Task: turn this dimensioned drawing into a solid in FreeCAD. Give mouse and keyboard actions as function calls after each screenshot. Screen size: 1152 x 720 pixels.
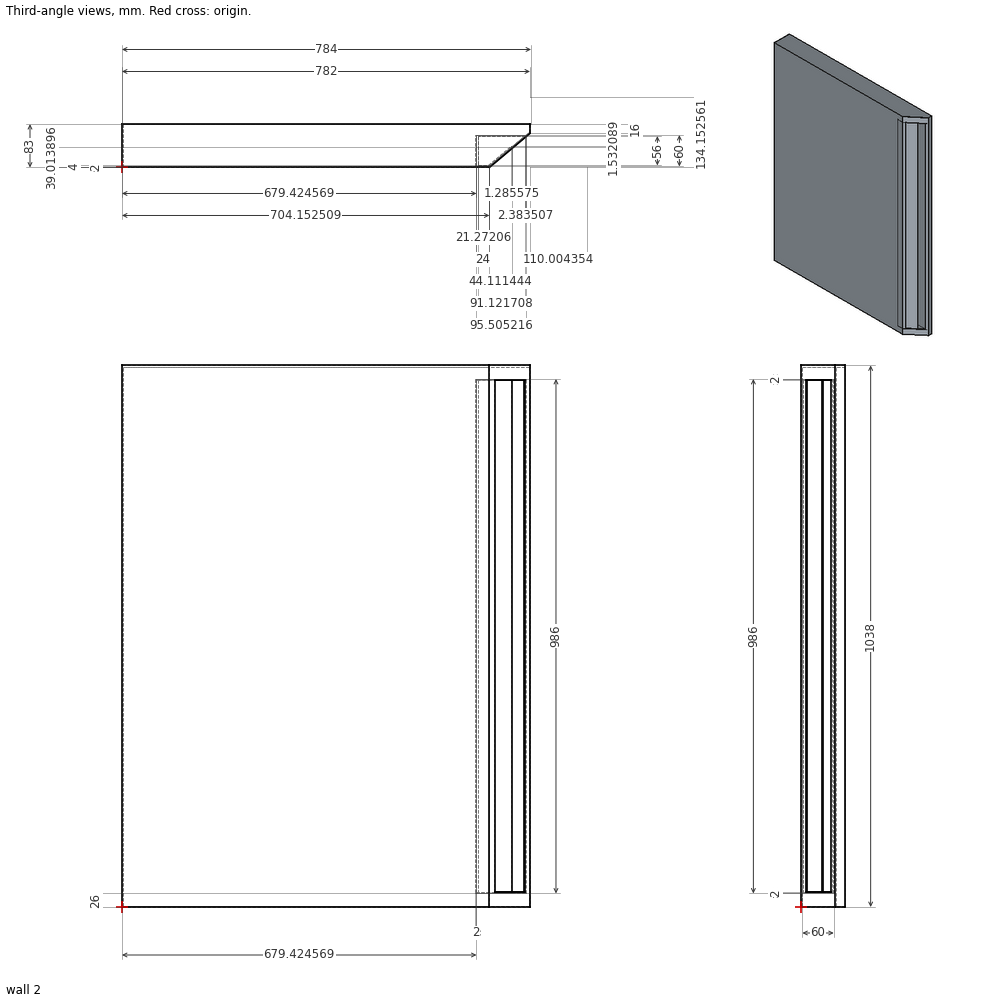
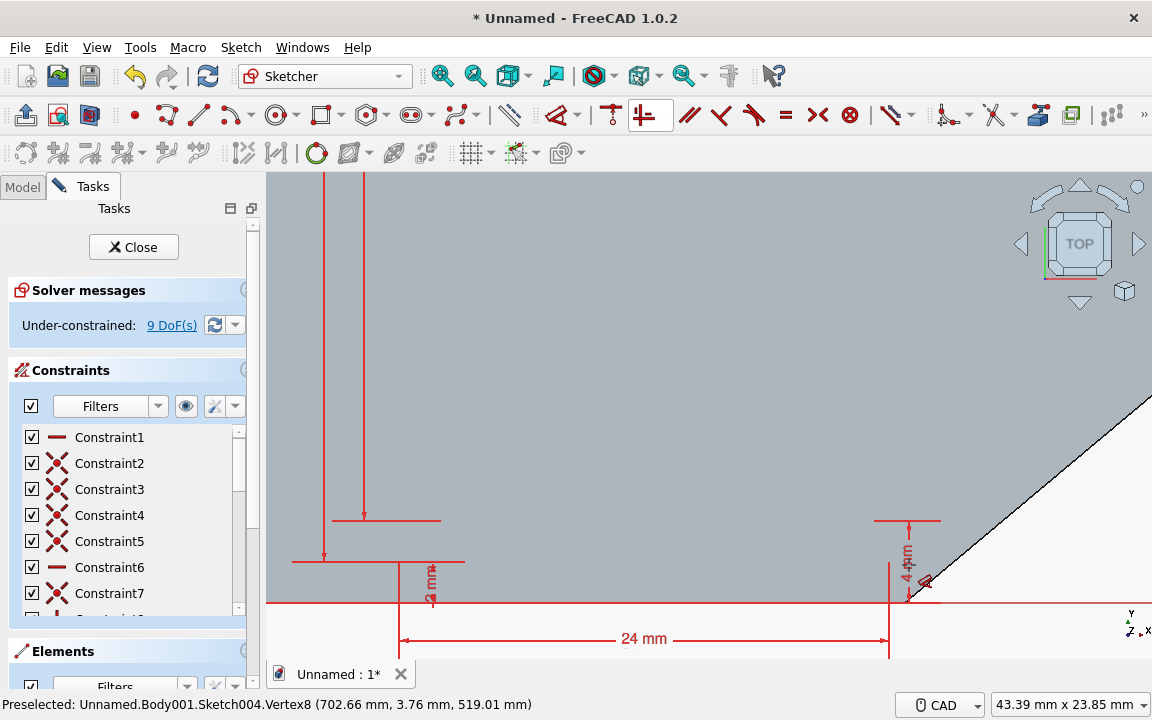
scroll(400, 568, down, 7)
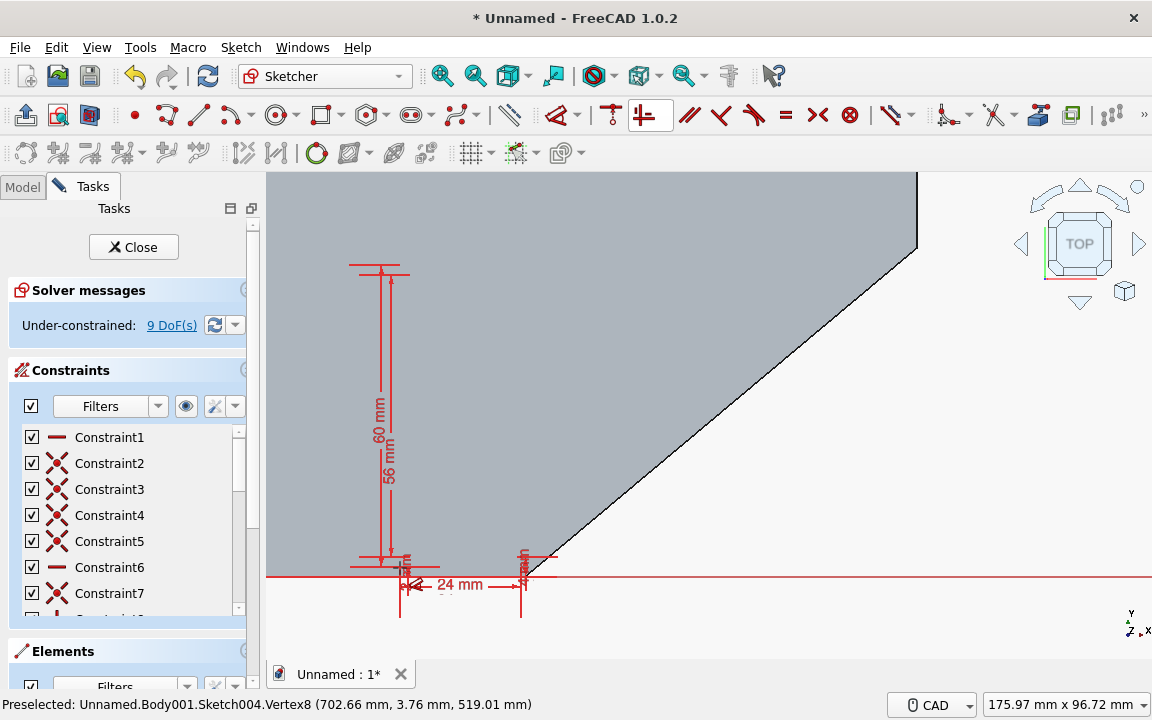
scroll(485, 557, up, 2)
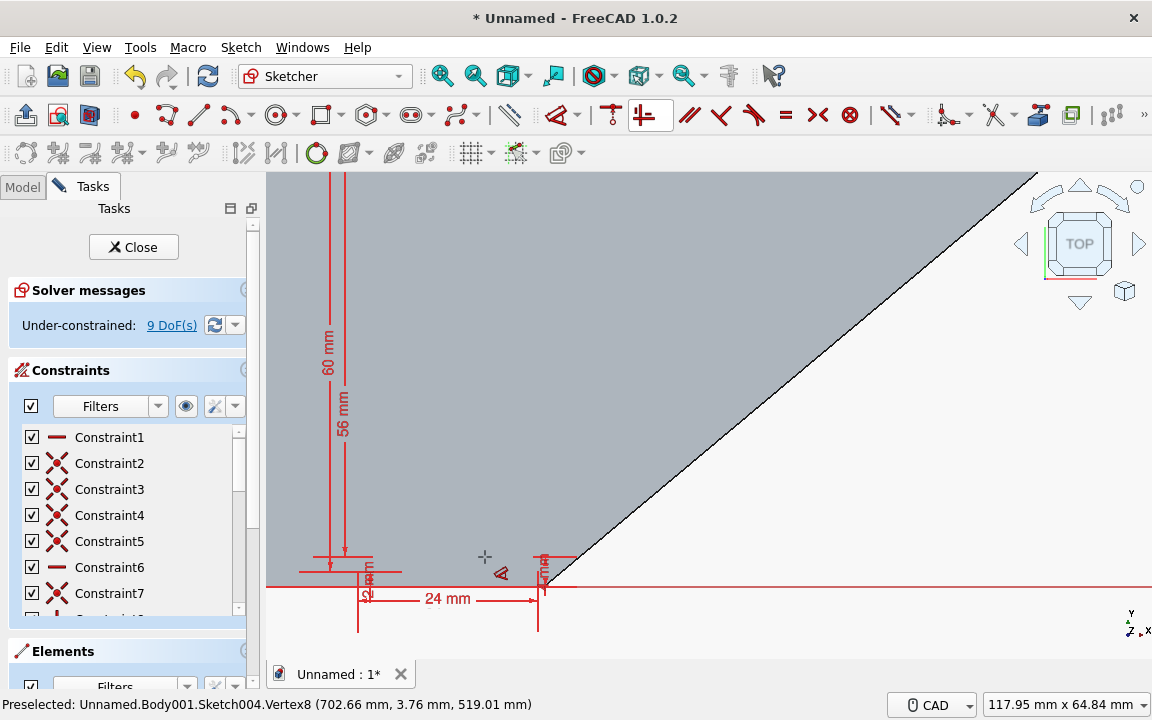
click(485, 557)
click(453, 523)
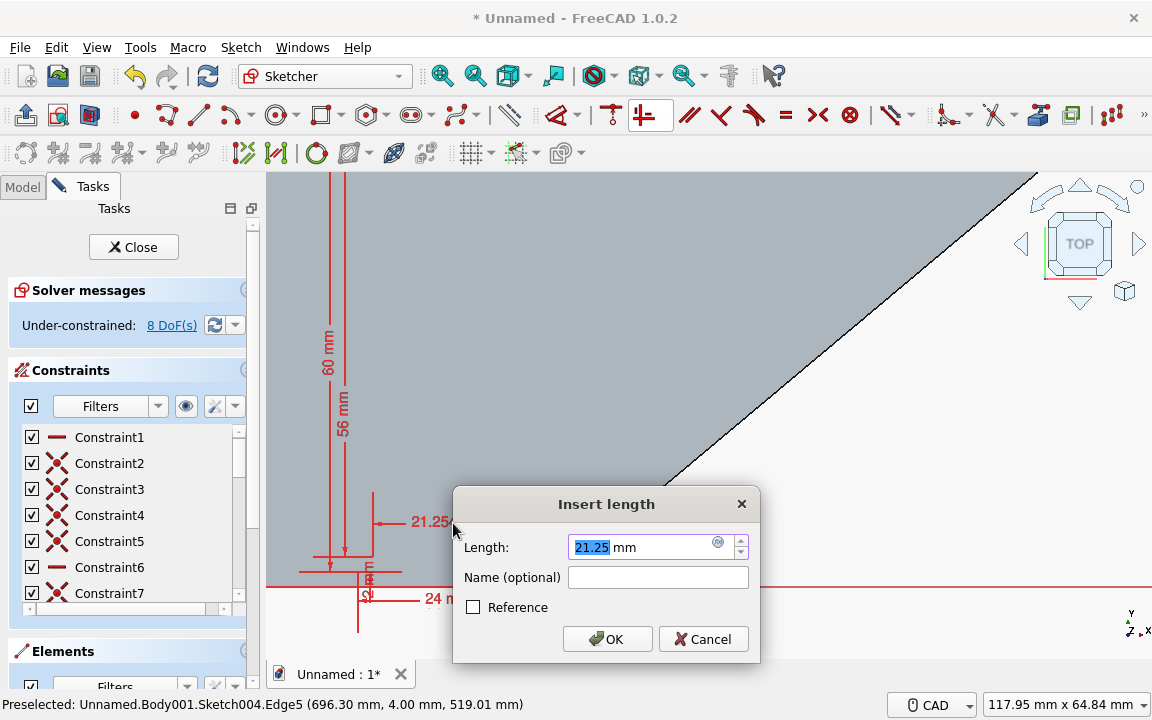
text(21.27206)
key(Return)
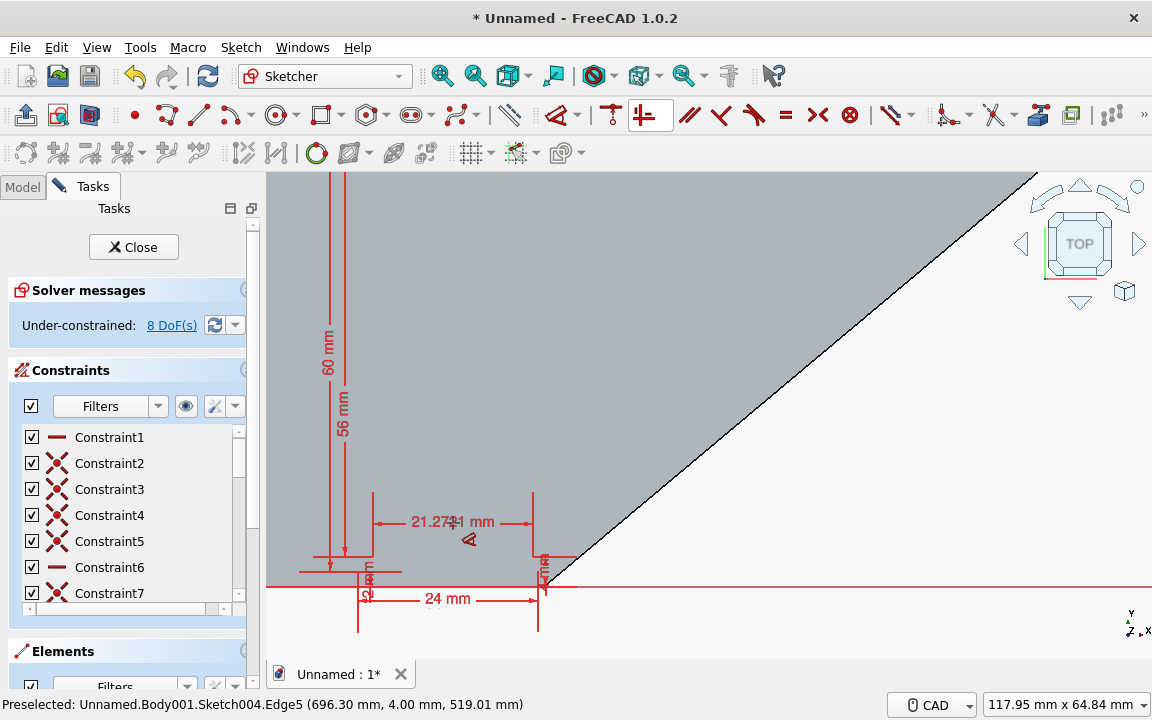
scroll(485, 556, down, 2)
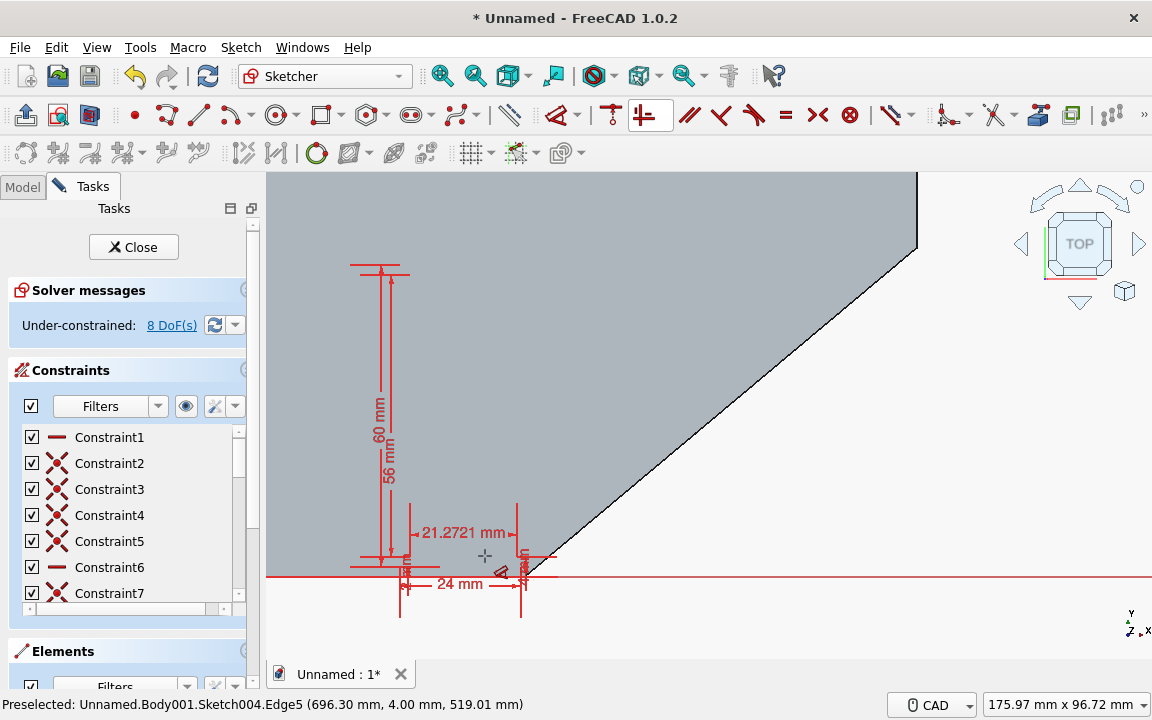
scroll(548, 275, up, 2)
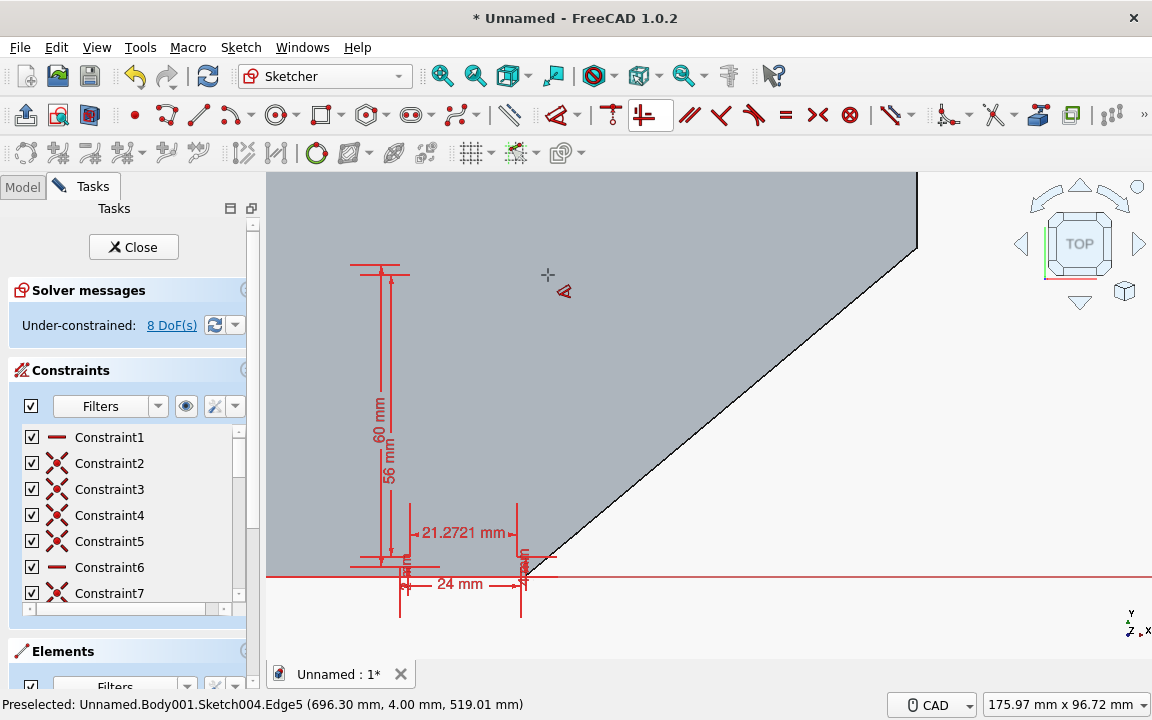
click(548, 275)
click(665, 241)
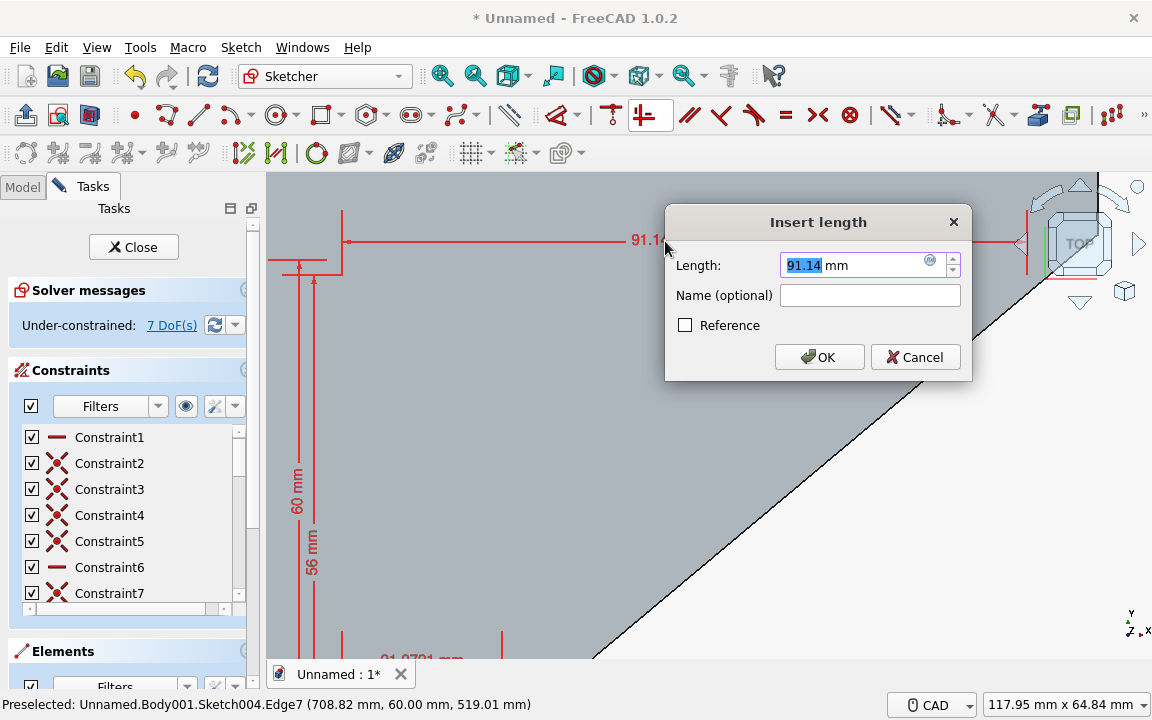
text(91.121708)
key(Return)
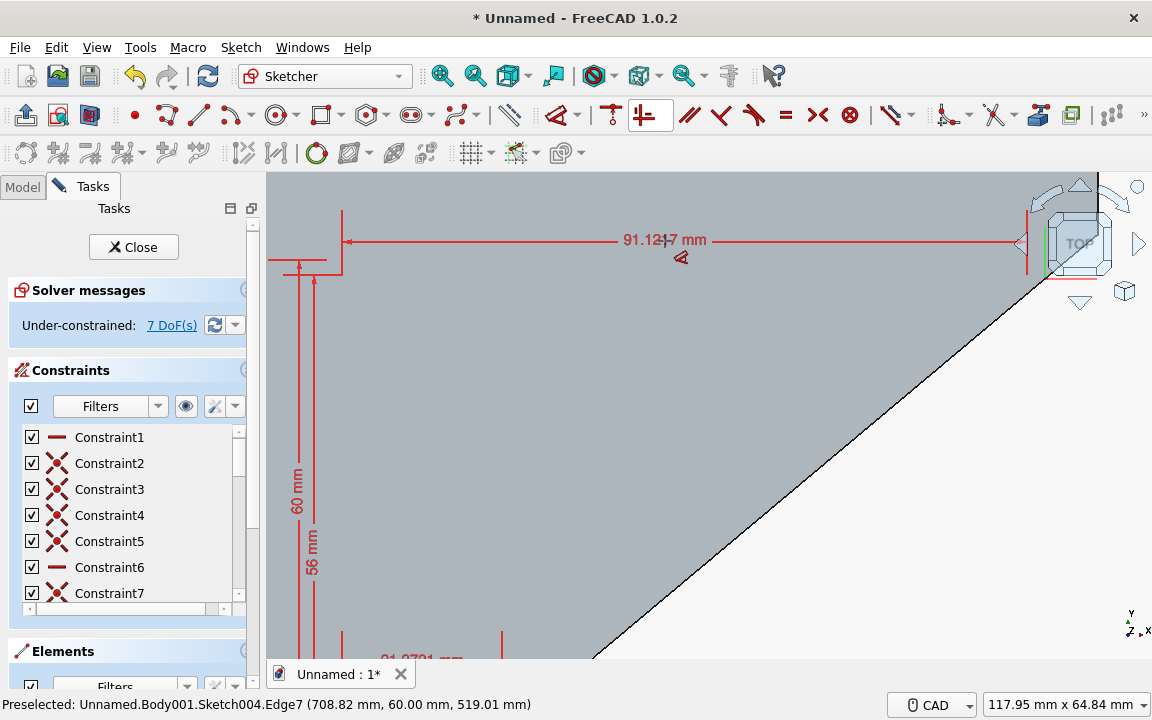
click(829, 260)
click(505, 226)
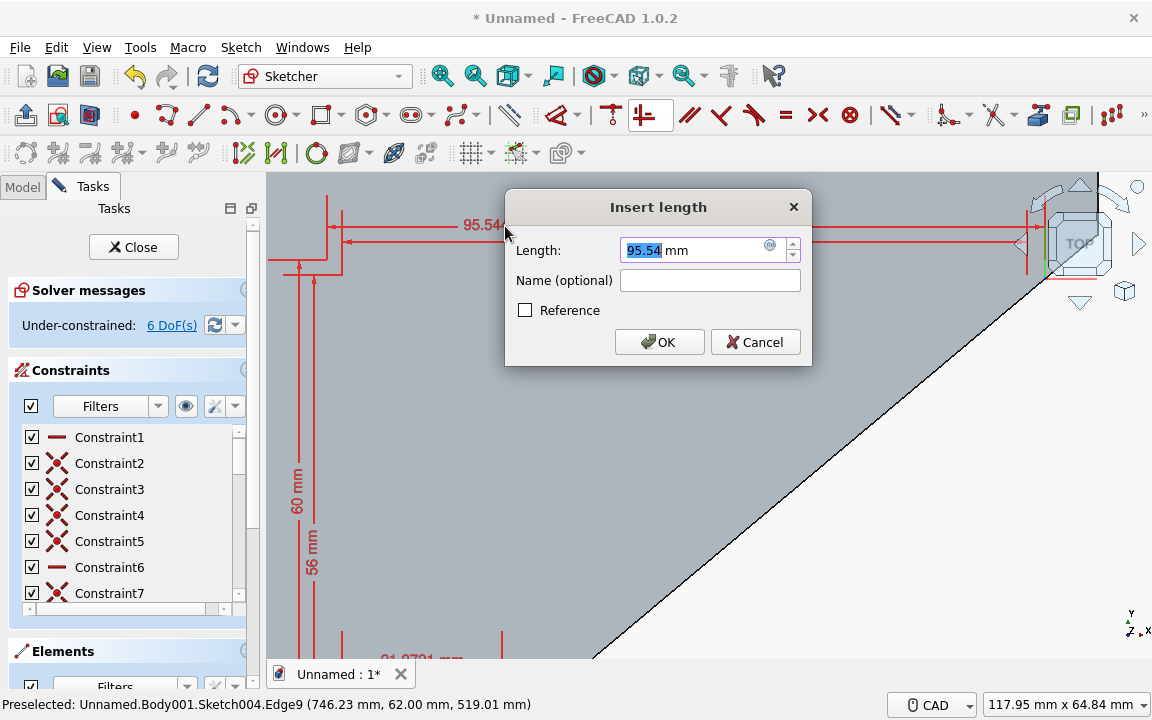
text(95.505216)
key(Return)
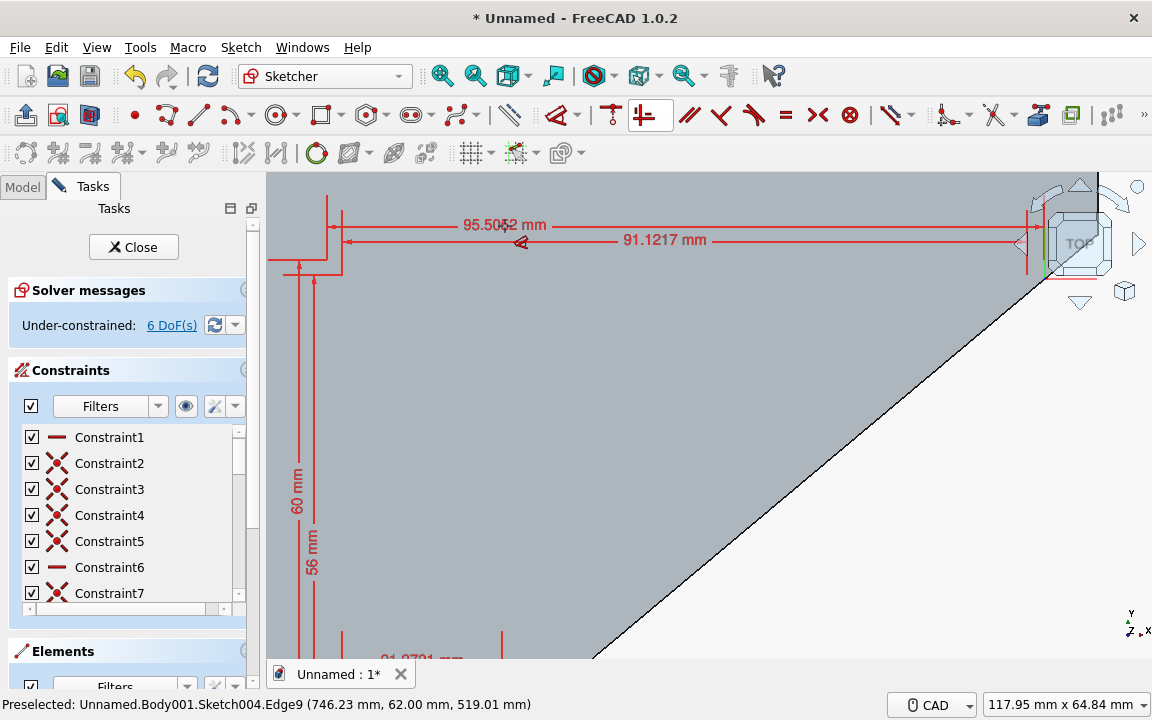
scroll(834, 428, up, 8)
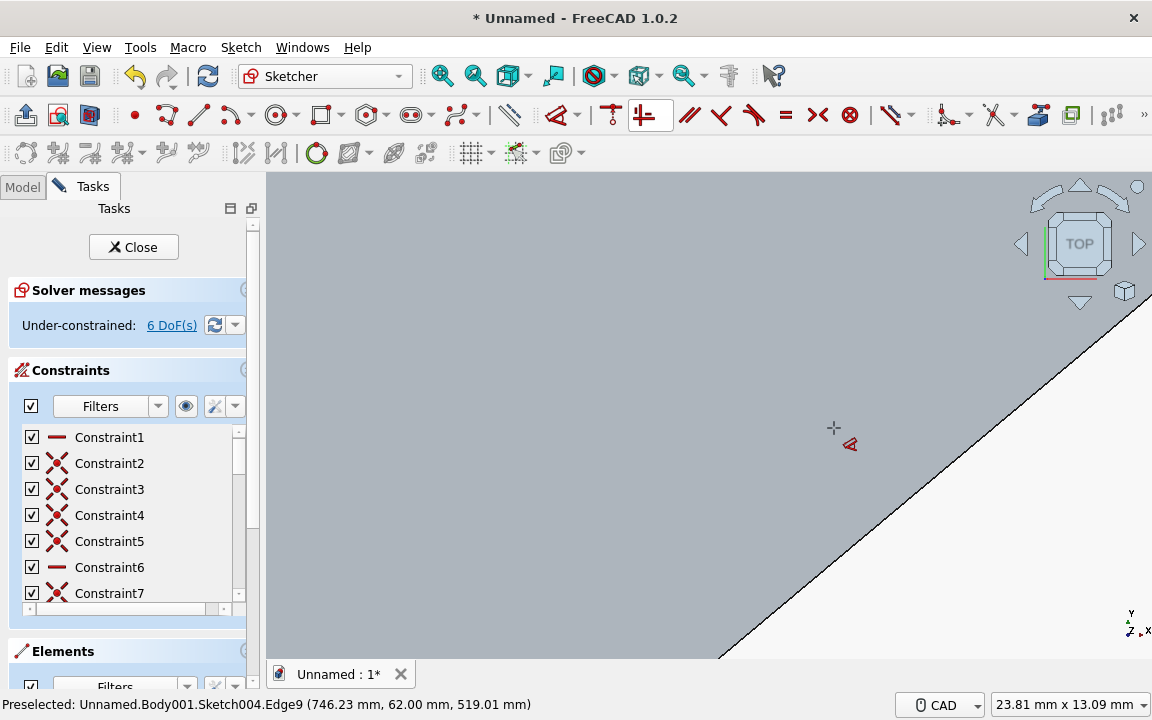
click(832, 425)
click(832, 361)